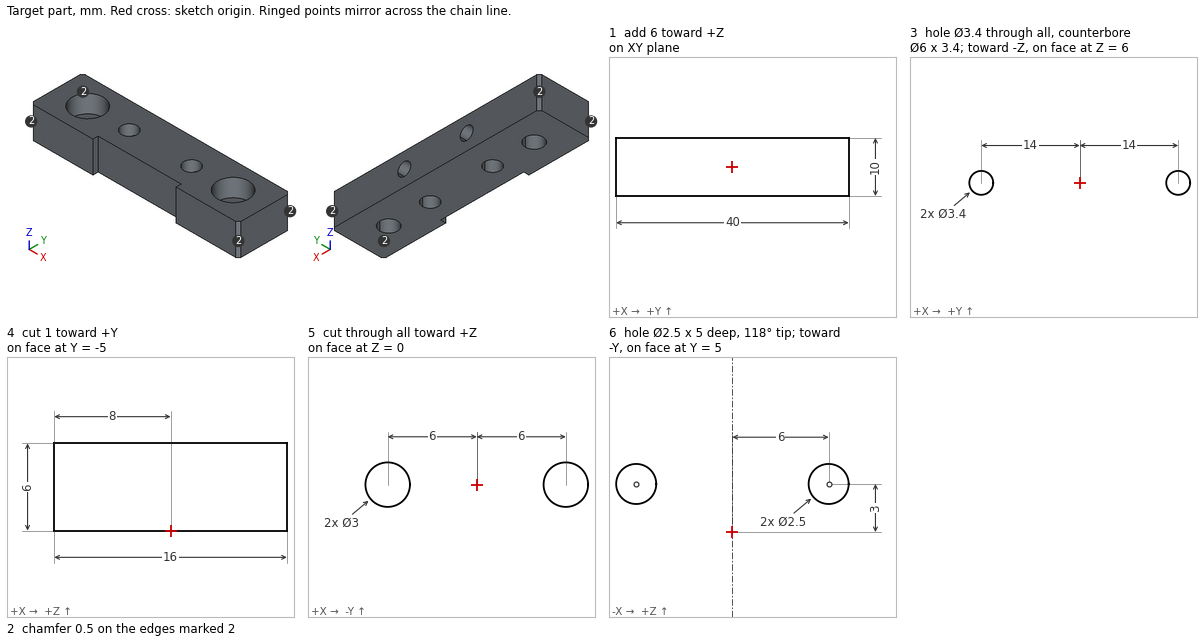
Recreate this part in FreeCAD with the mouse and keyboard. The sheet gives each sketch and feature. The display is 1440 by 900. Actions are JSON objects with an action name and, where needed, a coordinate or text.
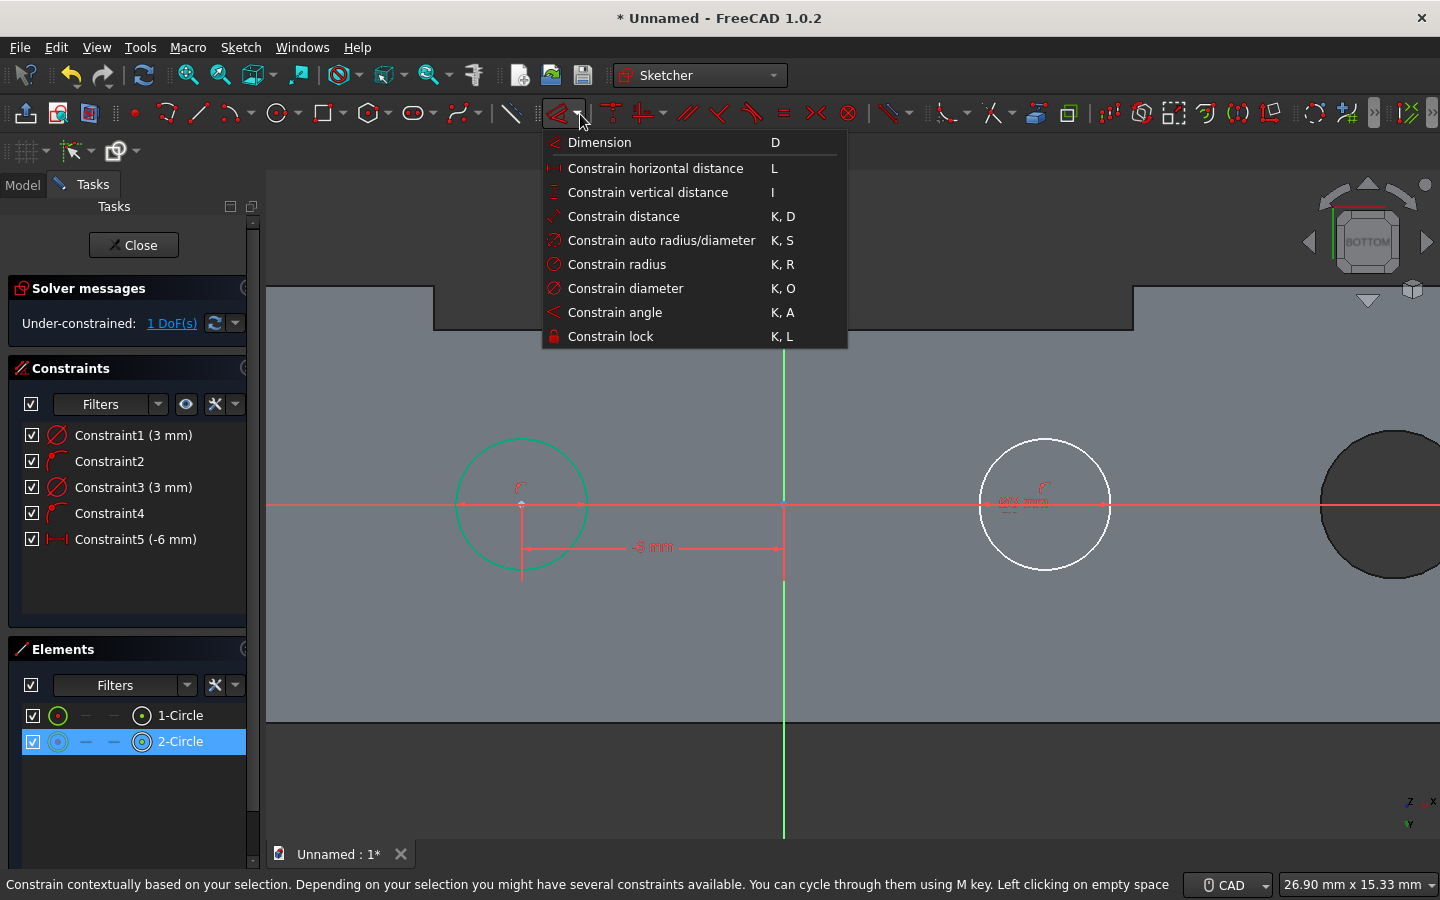
{"action": "left_click", "coordinate": [695, 168]}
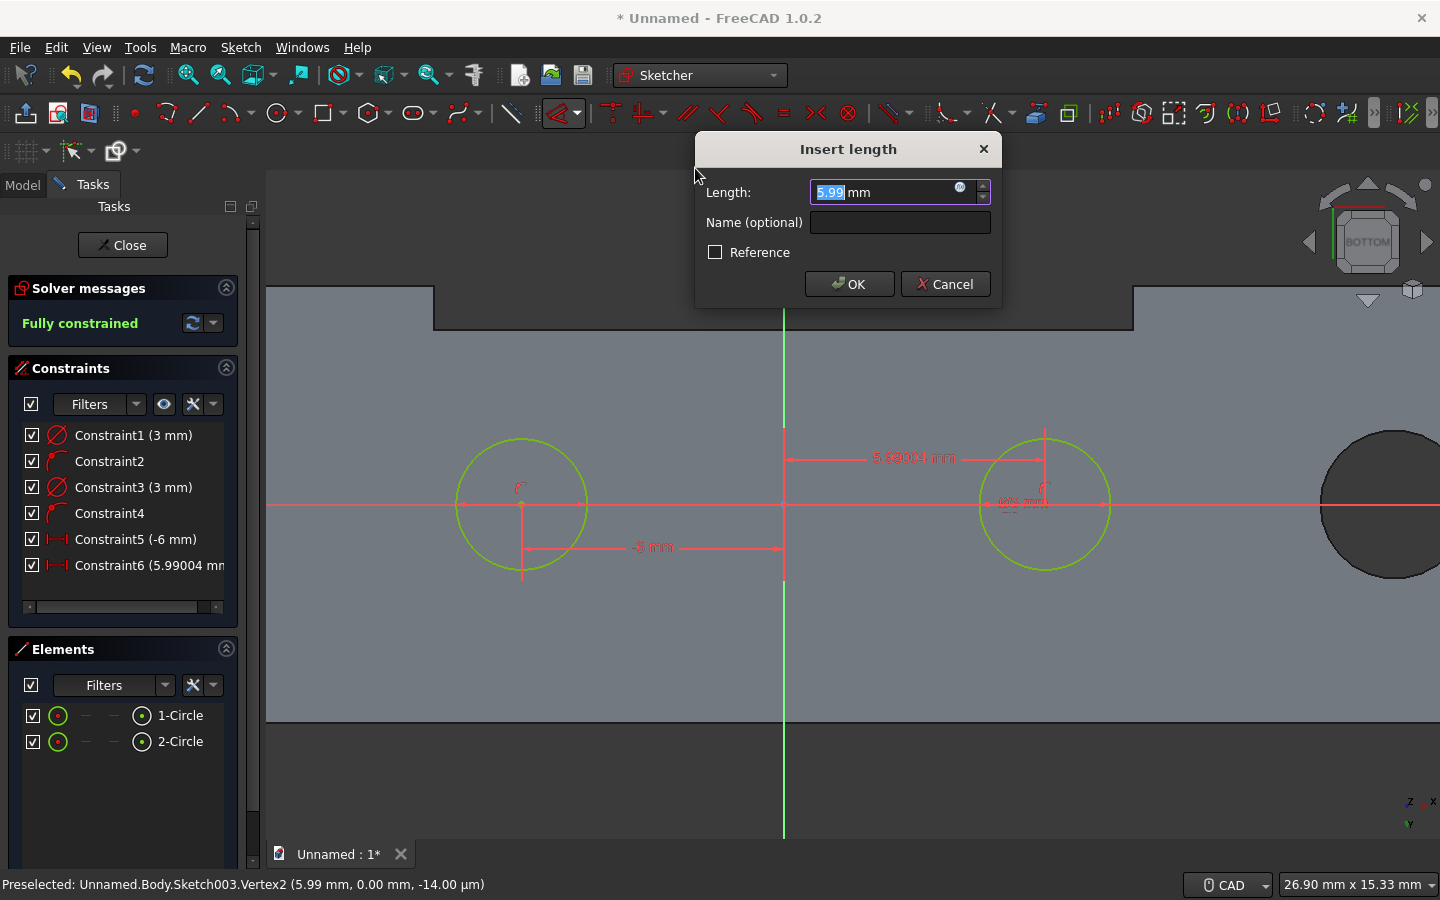
{"action": "type", "text": "6"}
{"action": "key", "text": "Return"}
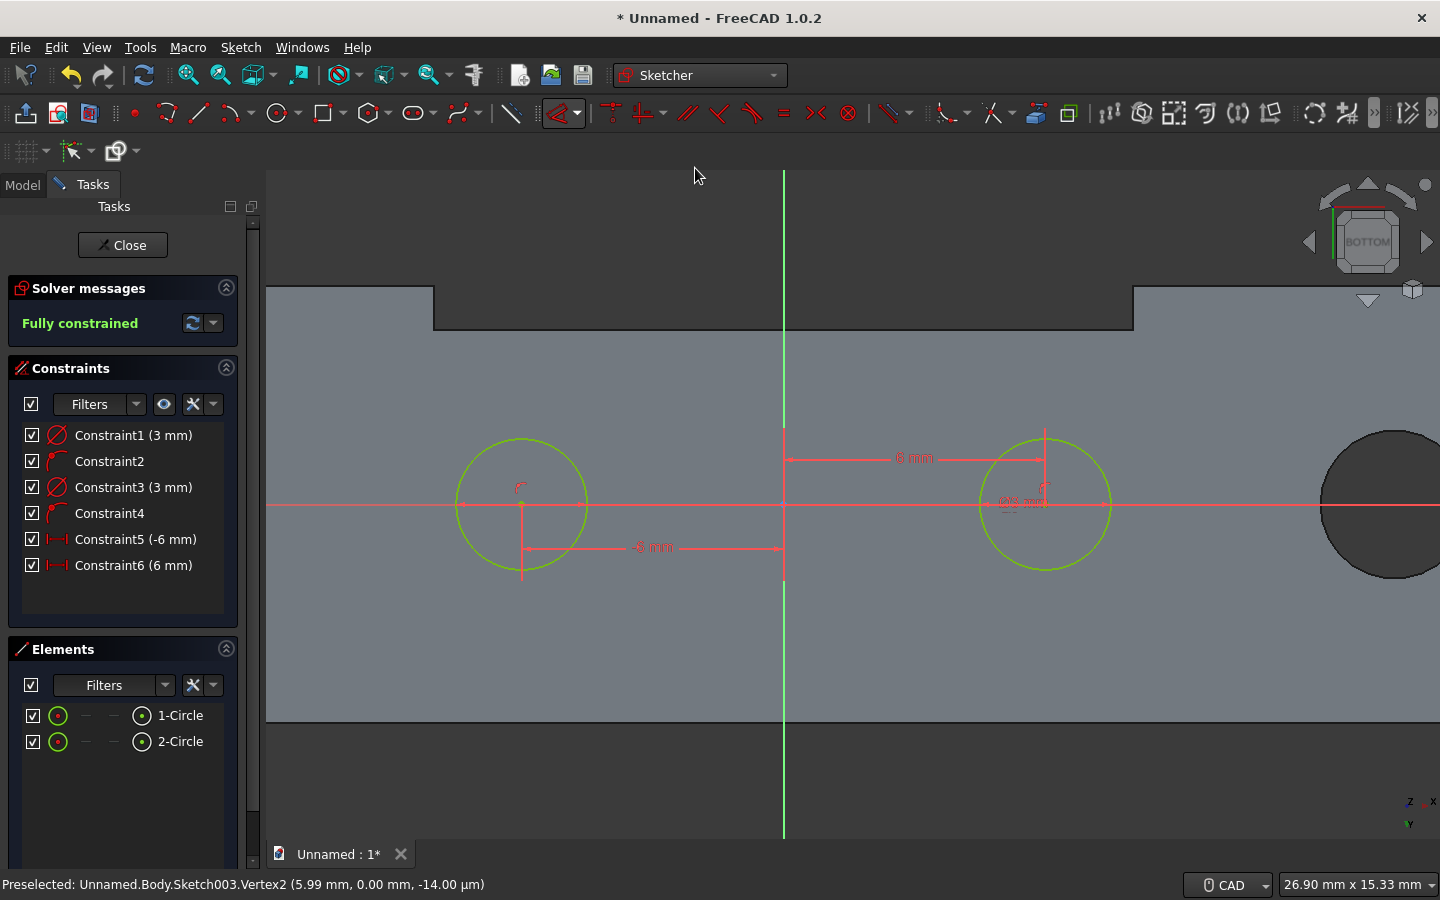
{"action": "left_click", "coordinate": [123, 245]}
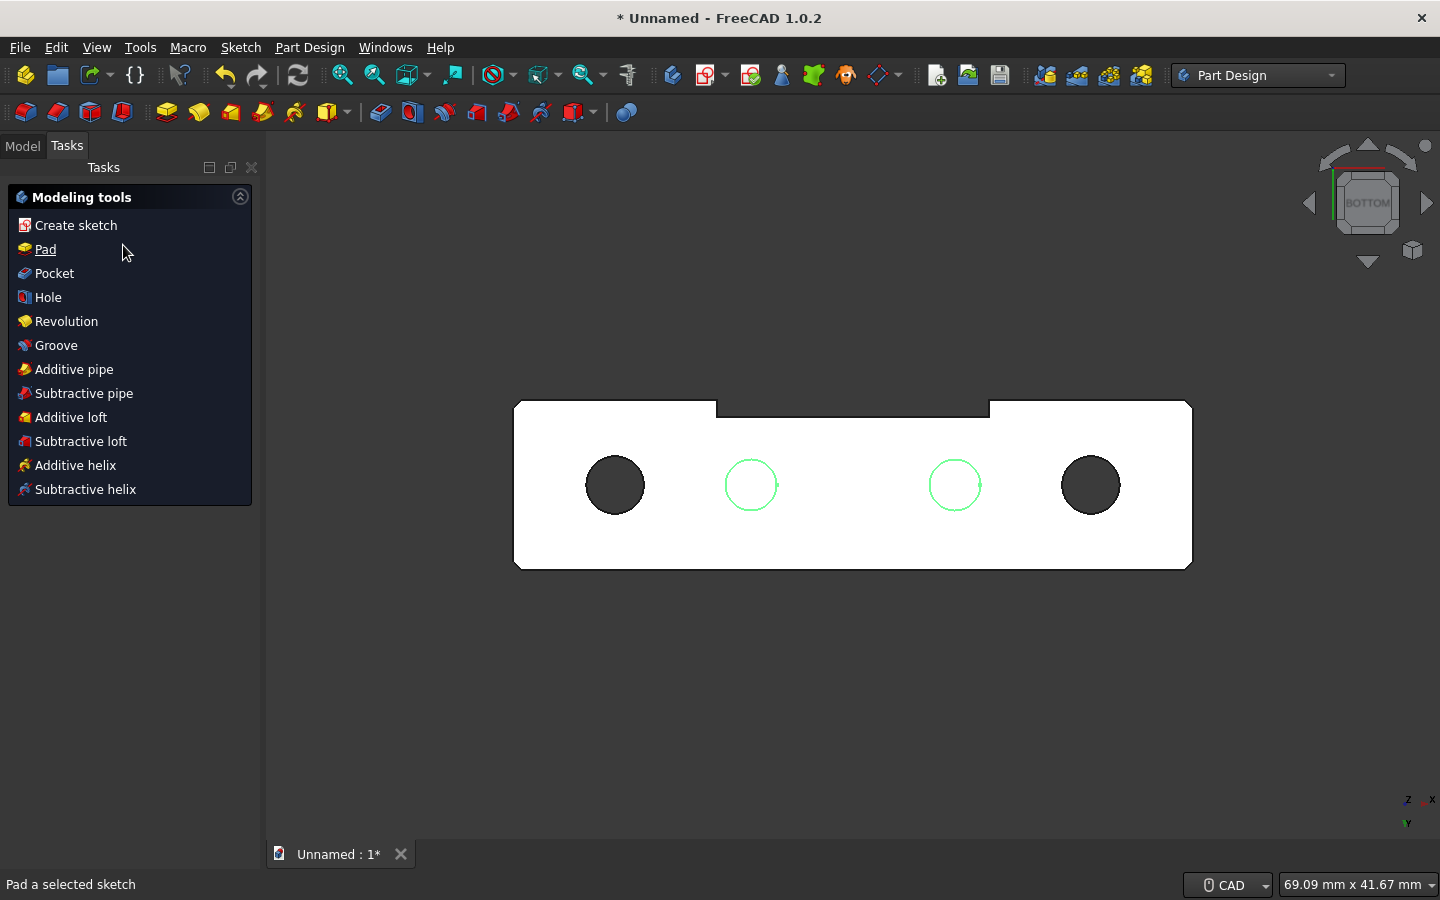
{"action": "left_click", "coordinate": [382, 112]}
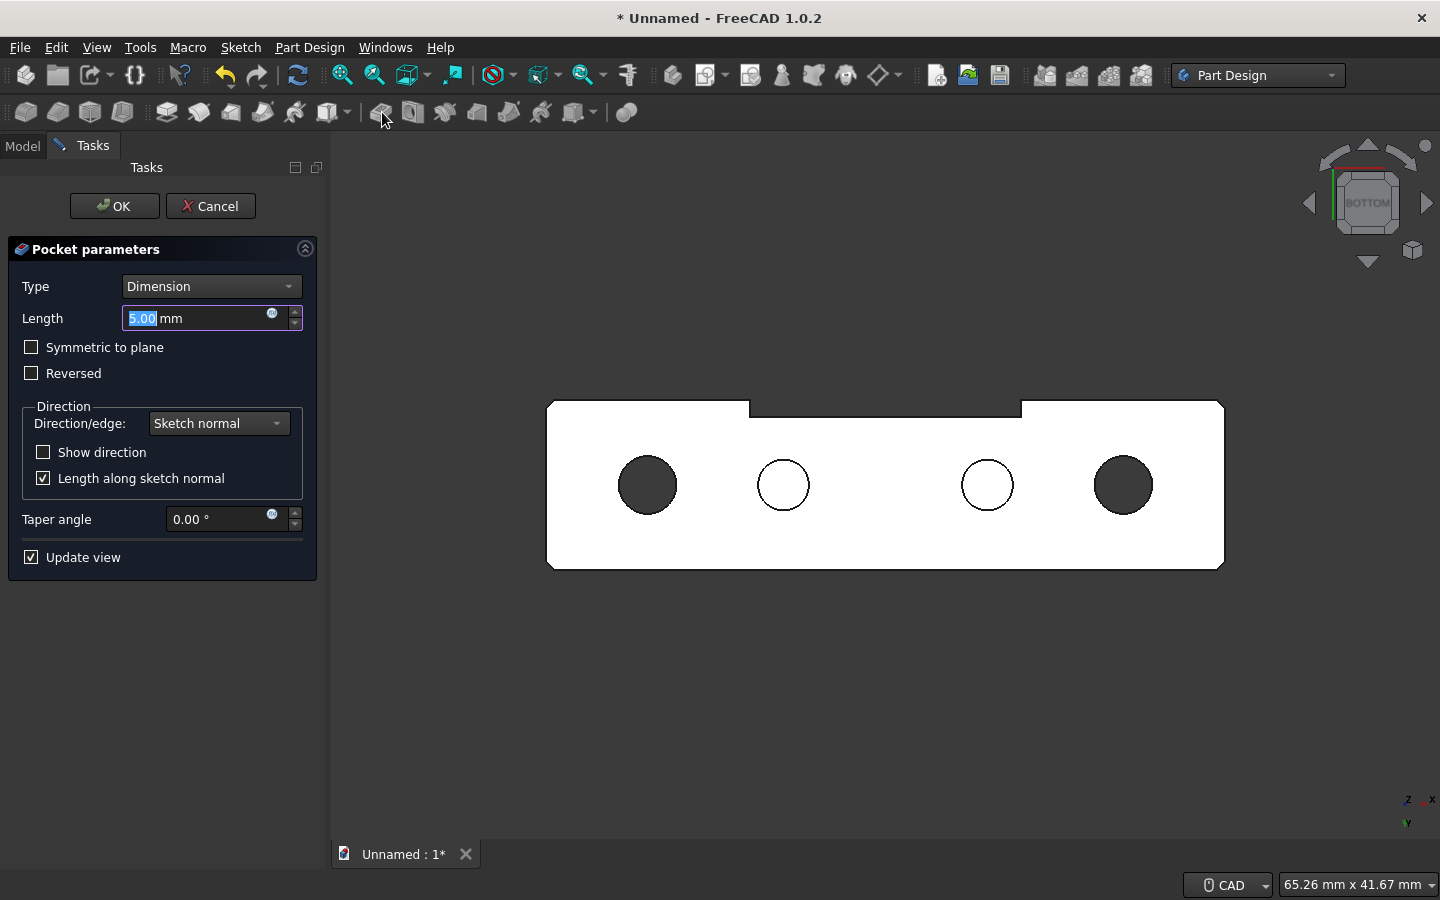
{"action": "left_click", "coordinate": [212, 286]}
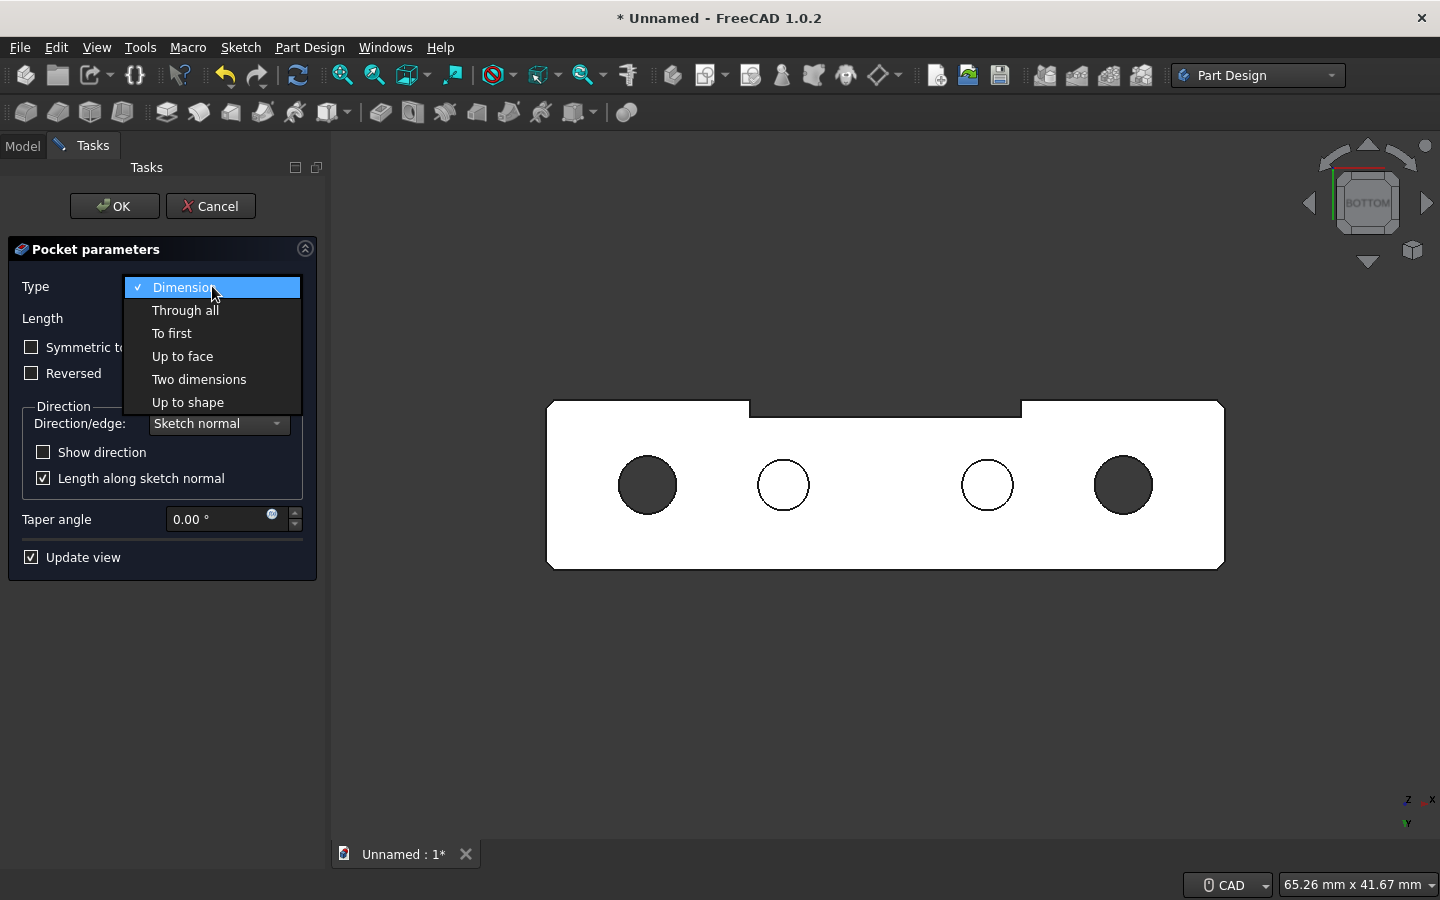
{"action": "left_click", "coordinate": [212, 310]}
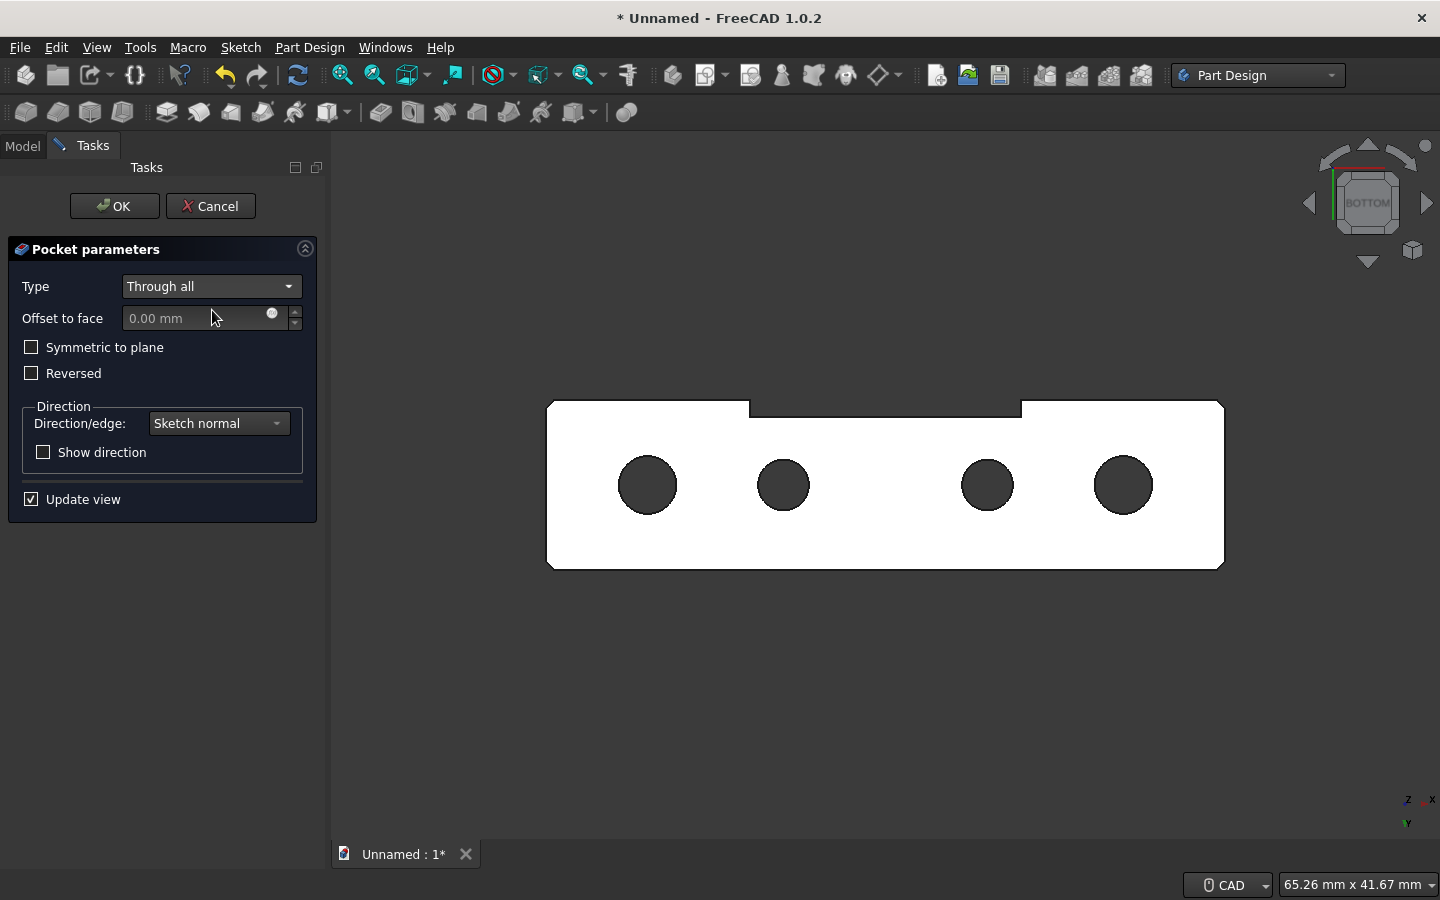
{"action": "left_click", "coordinate": [115, 206]}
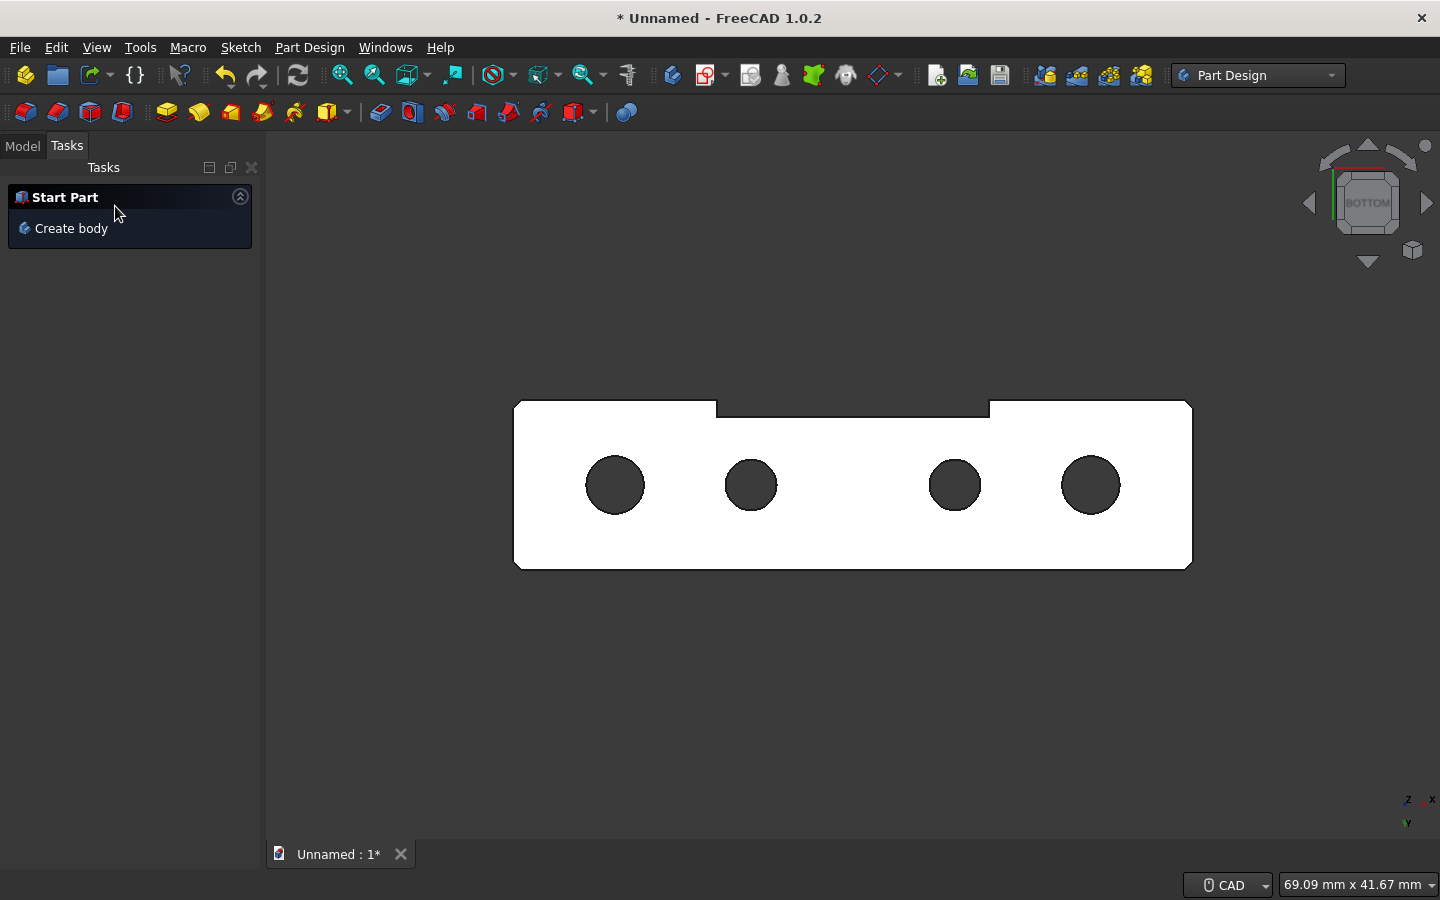
{"action": "key", "text": "4"}